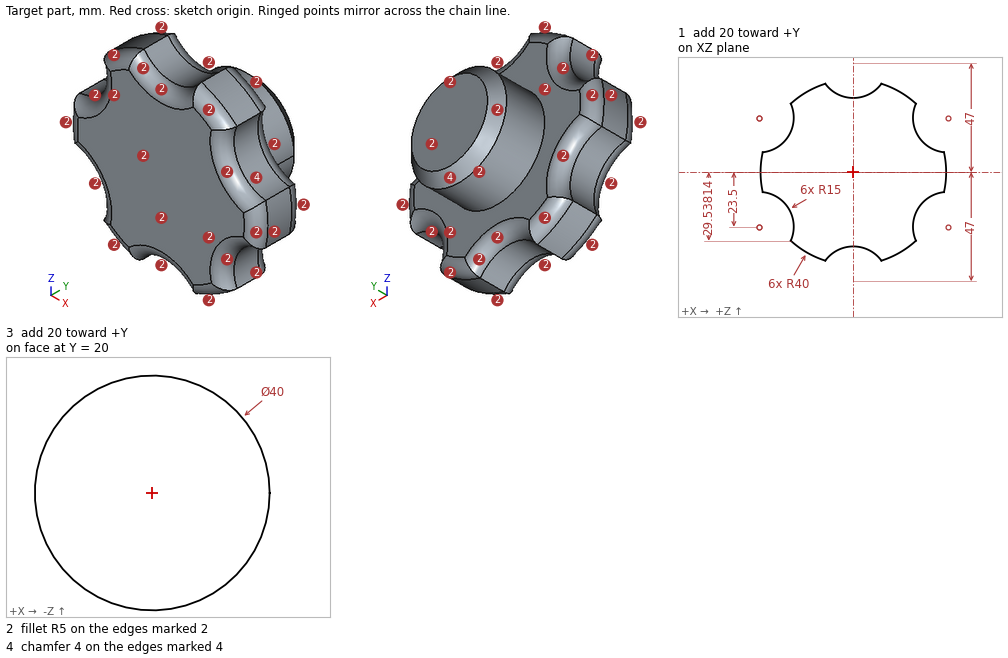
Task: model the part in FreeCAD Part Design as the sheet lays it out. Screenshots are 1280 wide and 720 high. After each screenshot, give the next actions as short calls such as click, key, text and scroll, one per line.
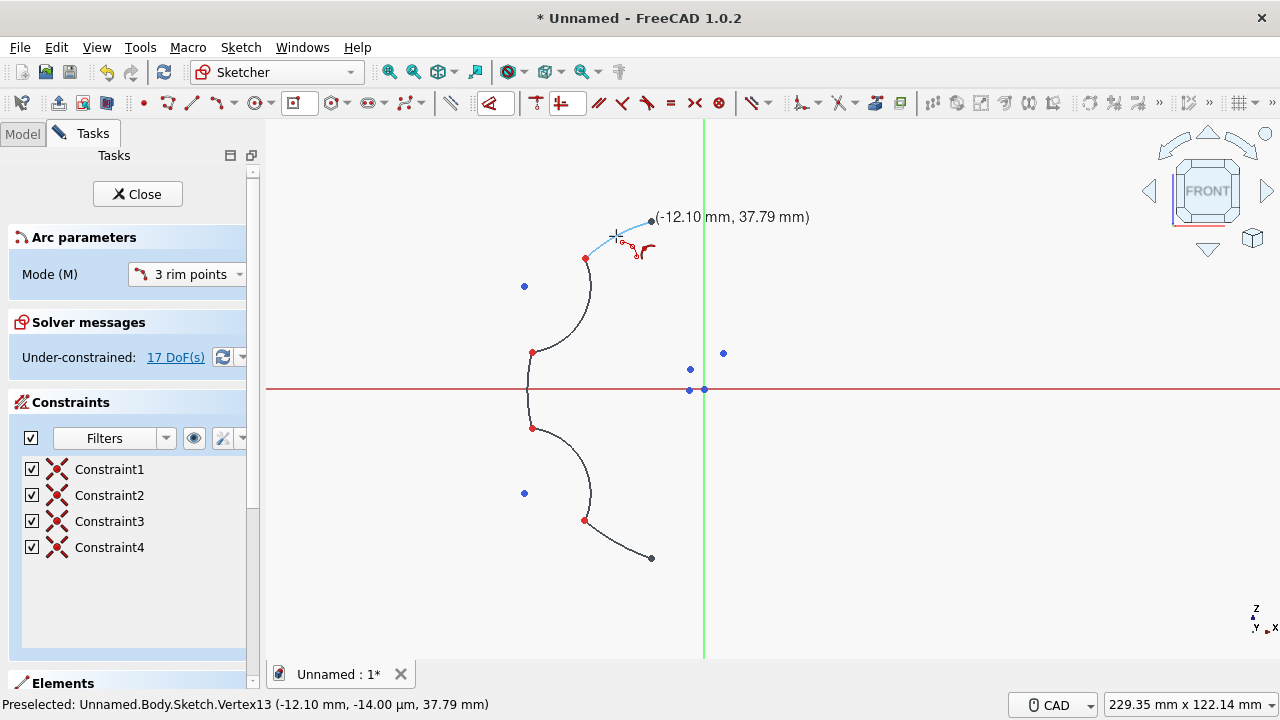
click(758, 221)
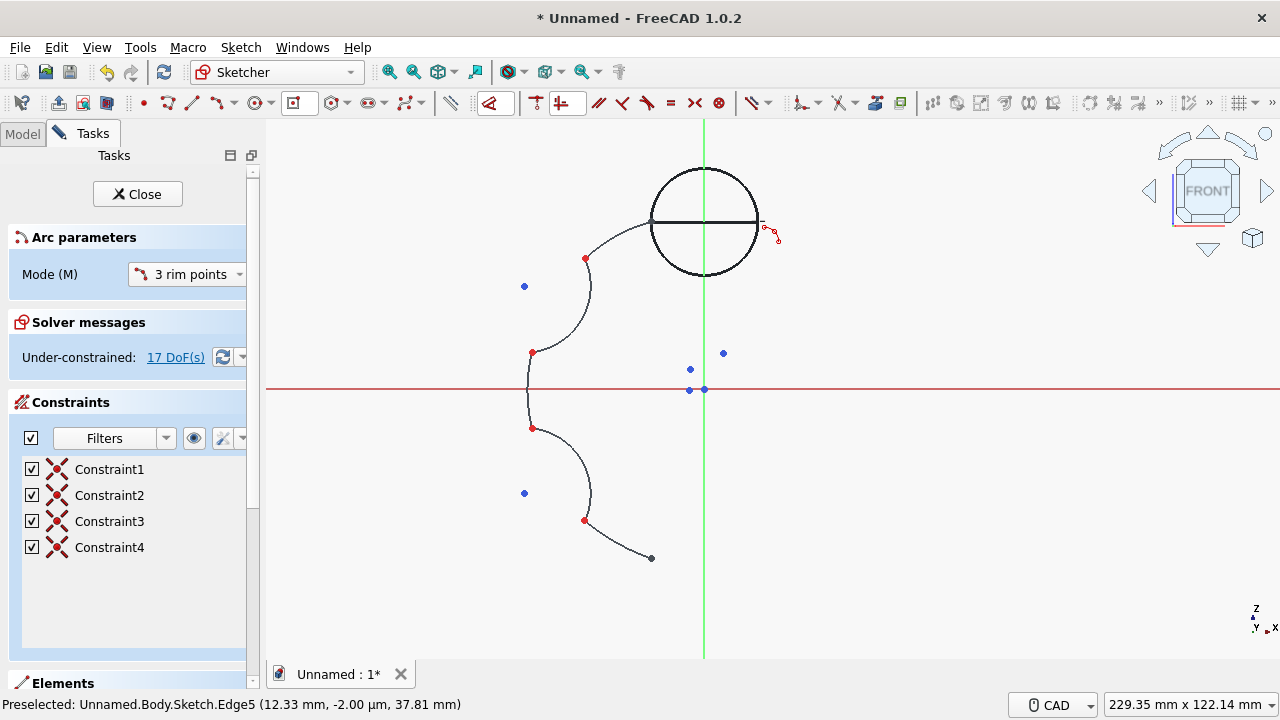
scroll(692, 246, up, 2)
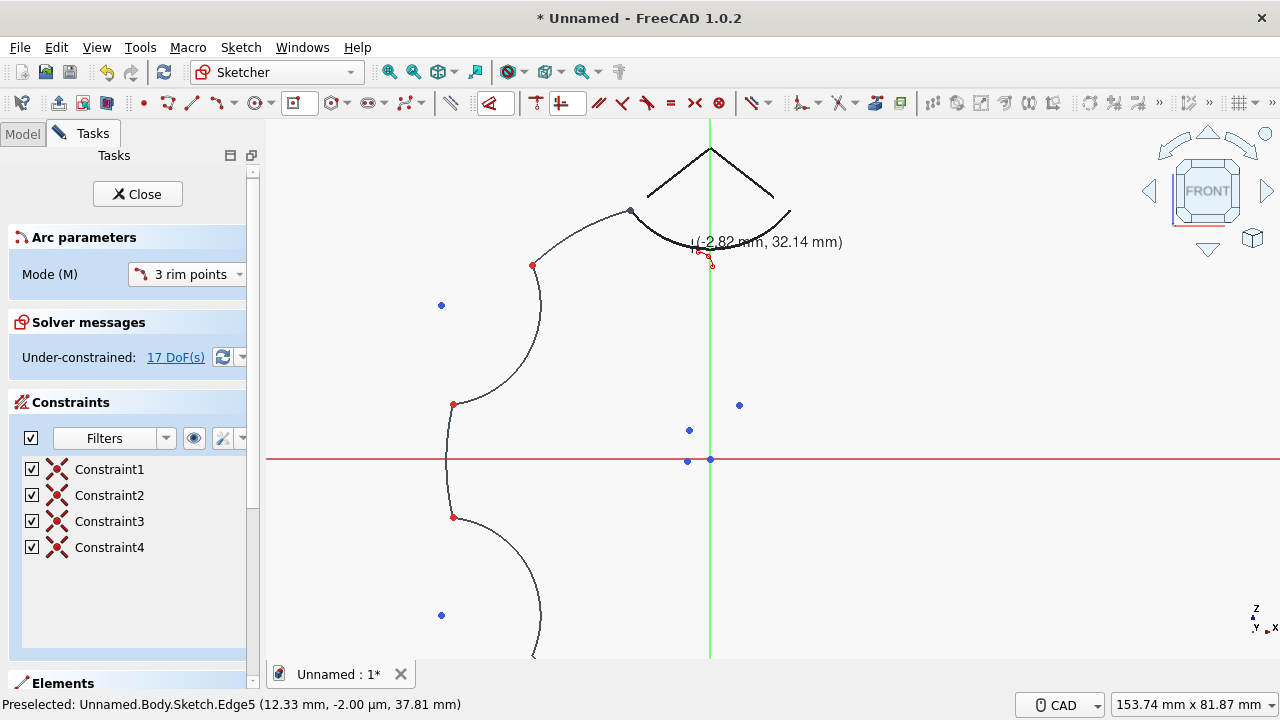
click(692, 247)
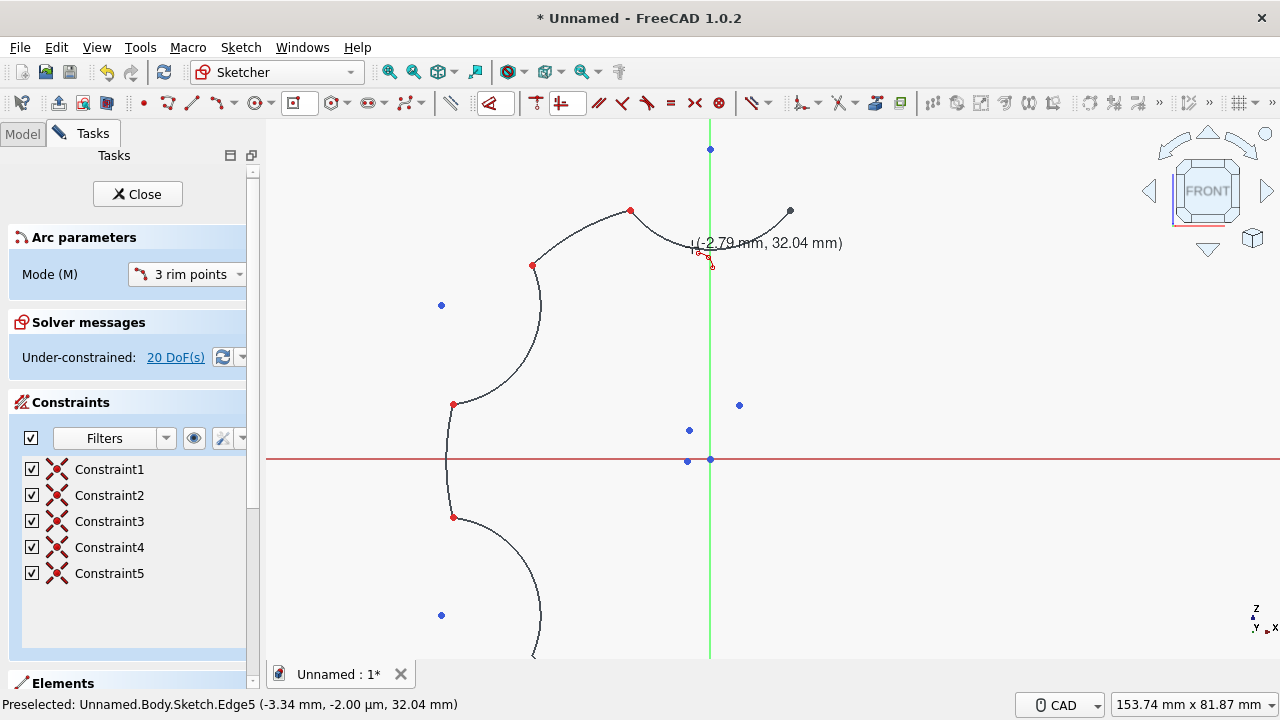
click(790, 210)
click(888, 265)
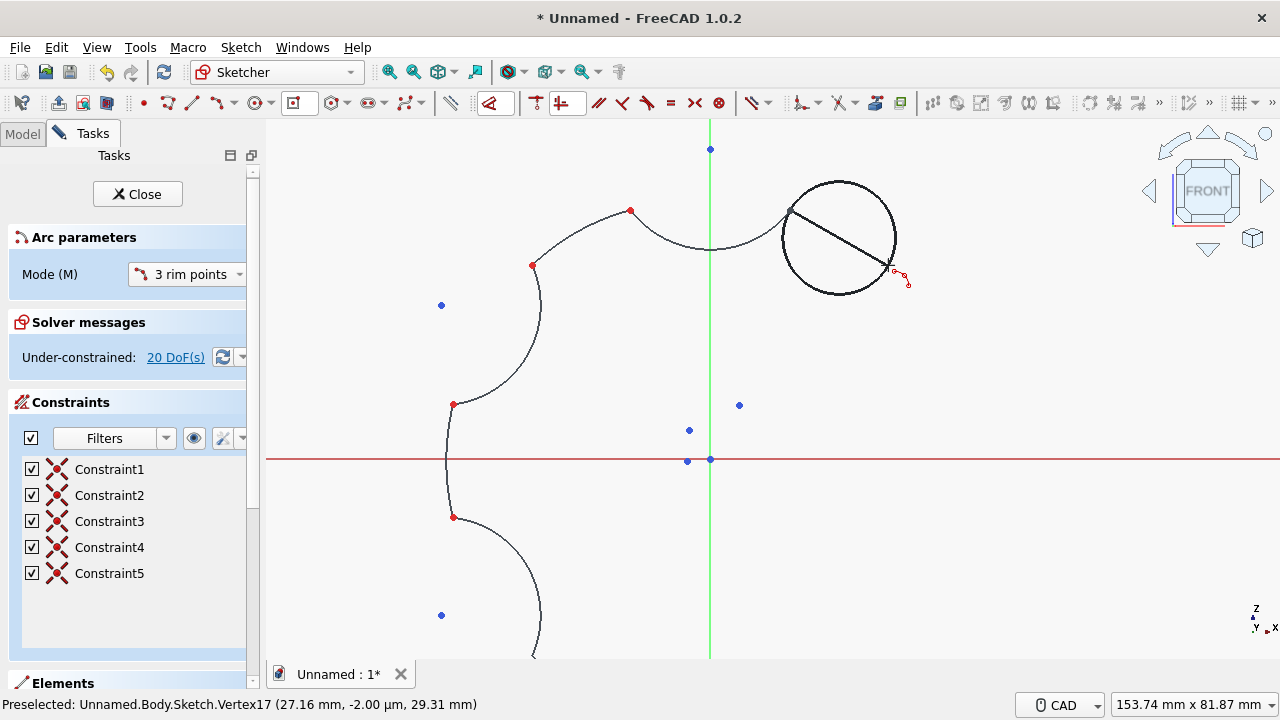
scroll(842, 231, up, 5)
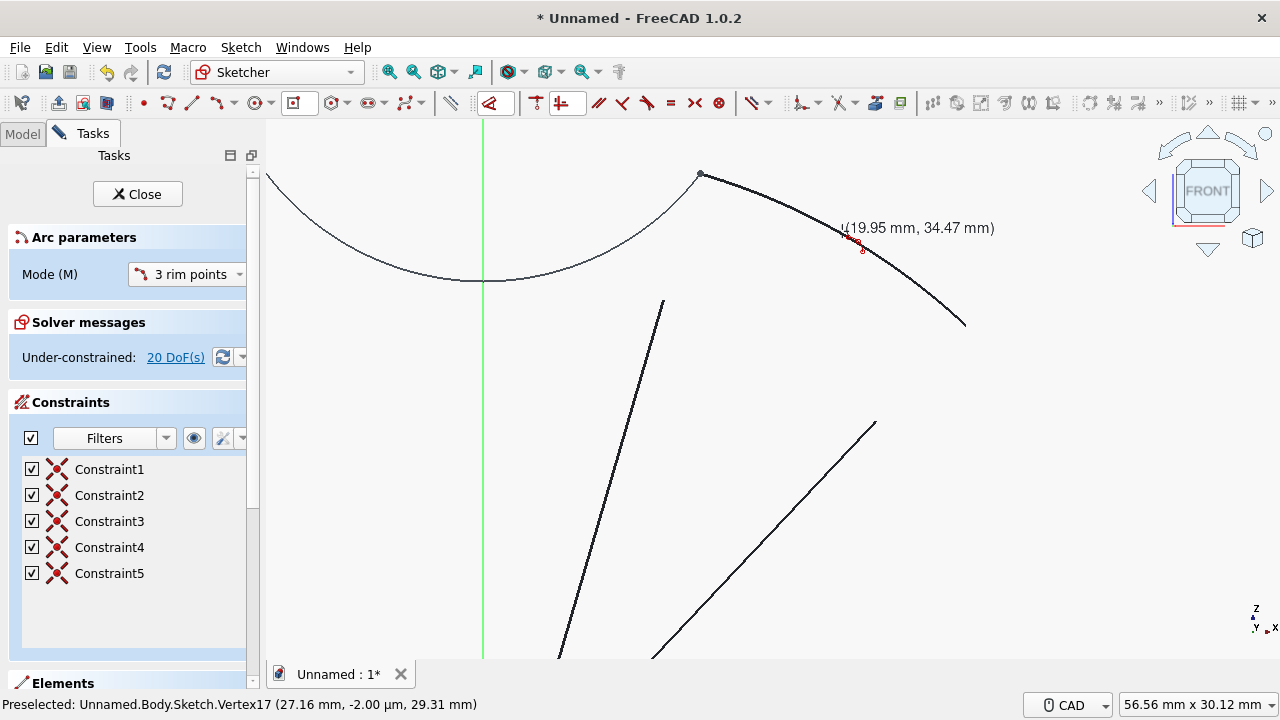
click(842, 230)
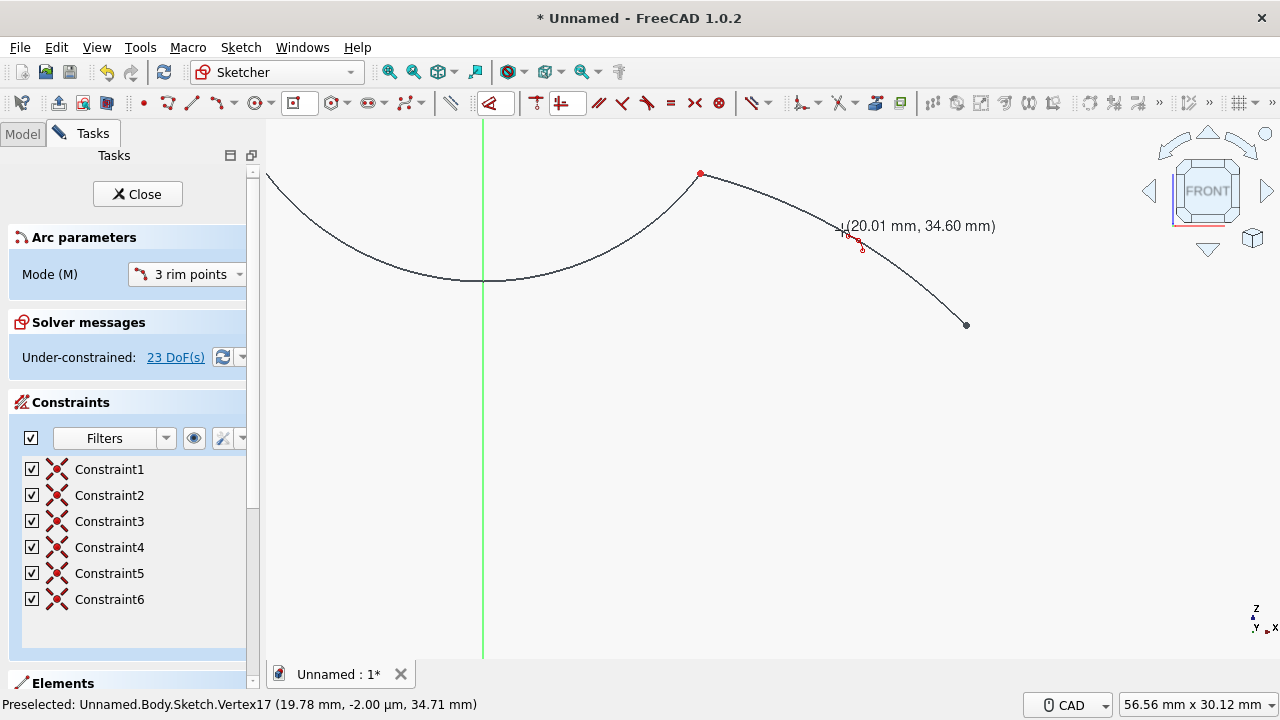
click(966, 326)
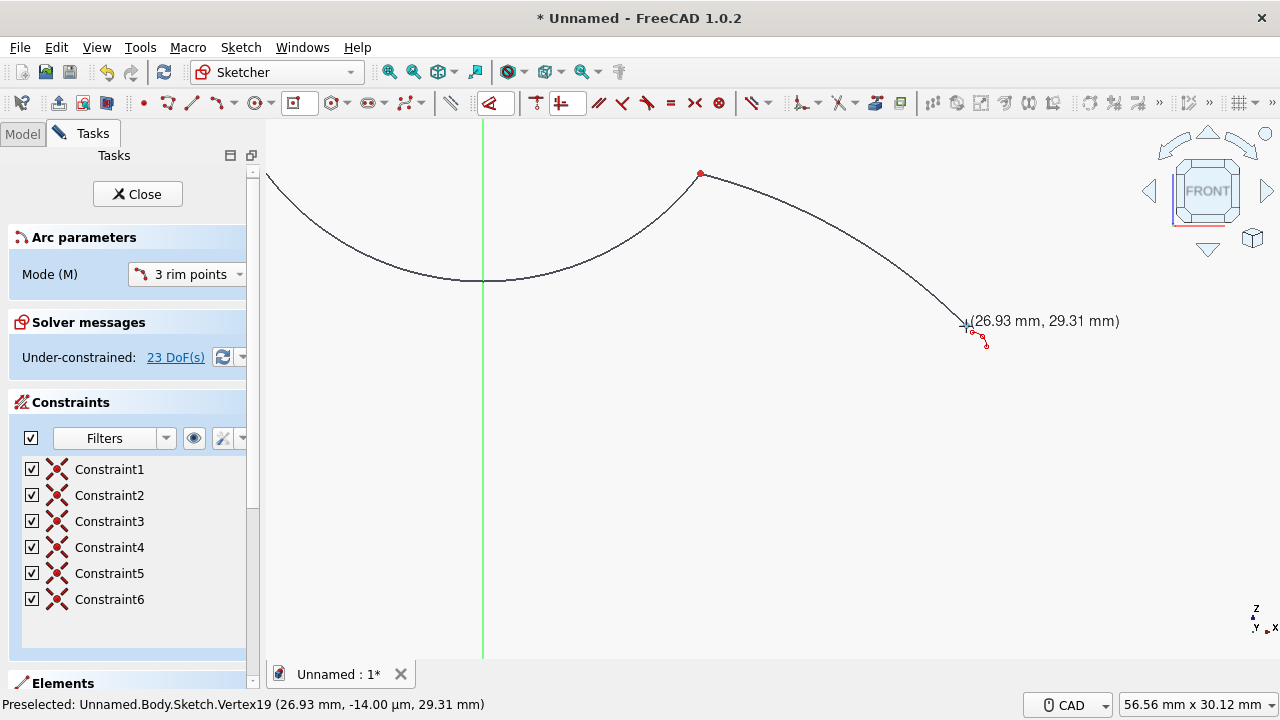
scroll(777, 238, down, 7)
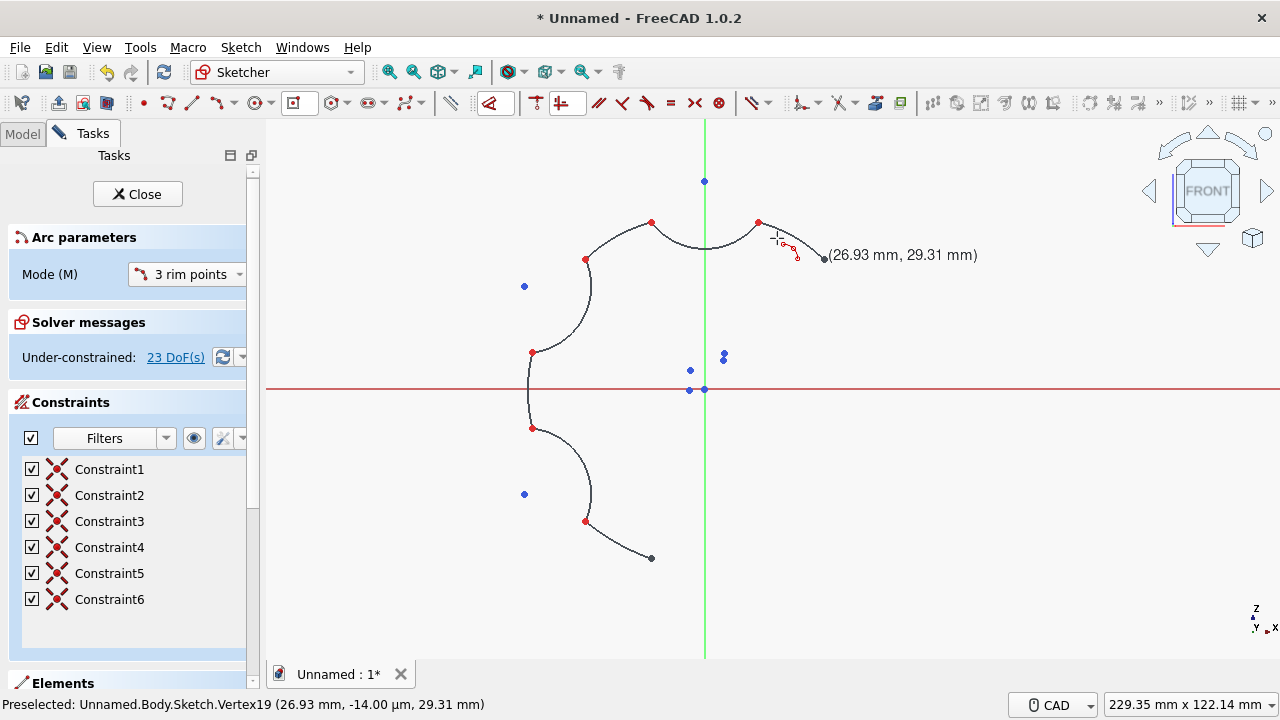
click(878, 351)
click(827, 319)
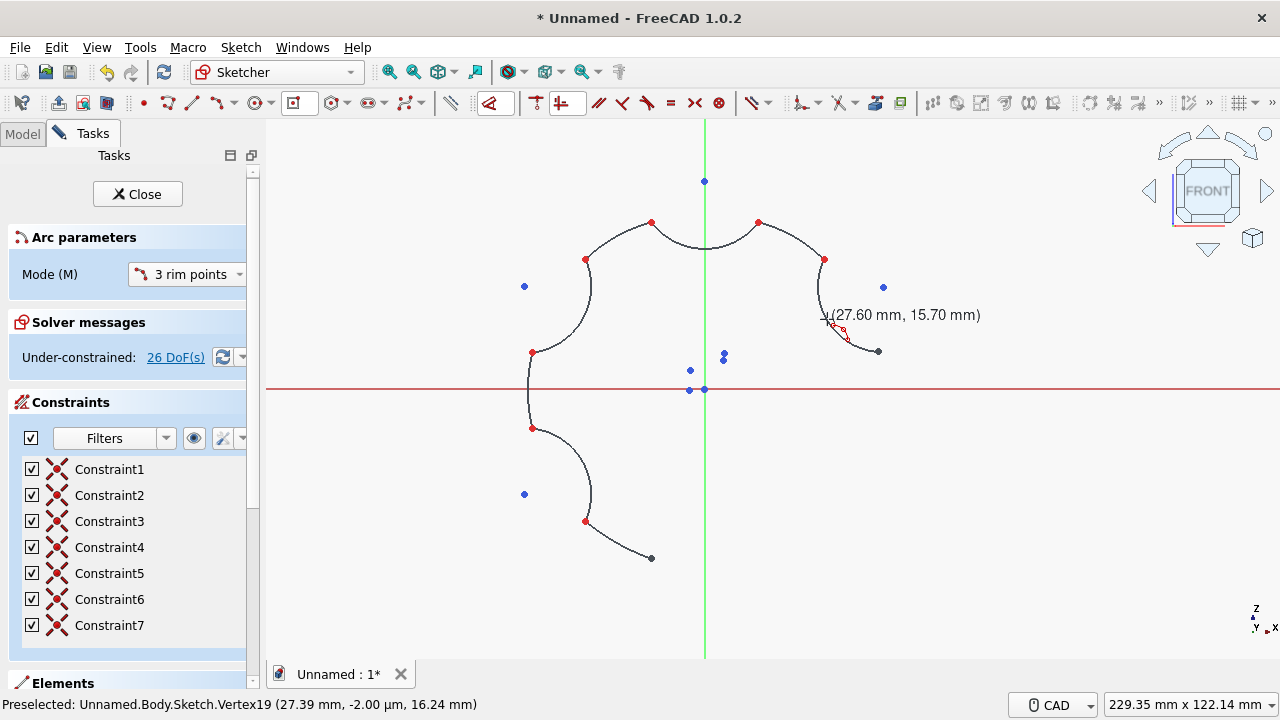
click(878, 352)
click(878, 427)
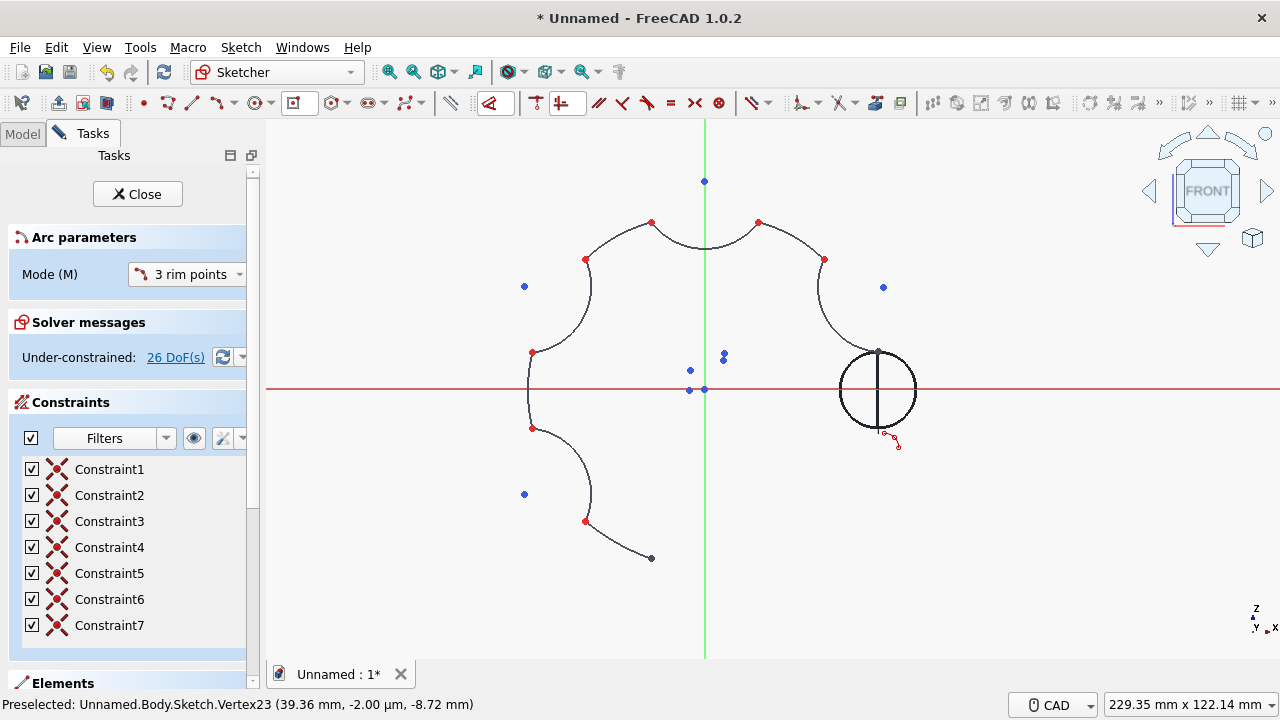
scroll(882, 397, up, 7)